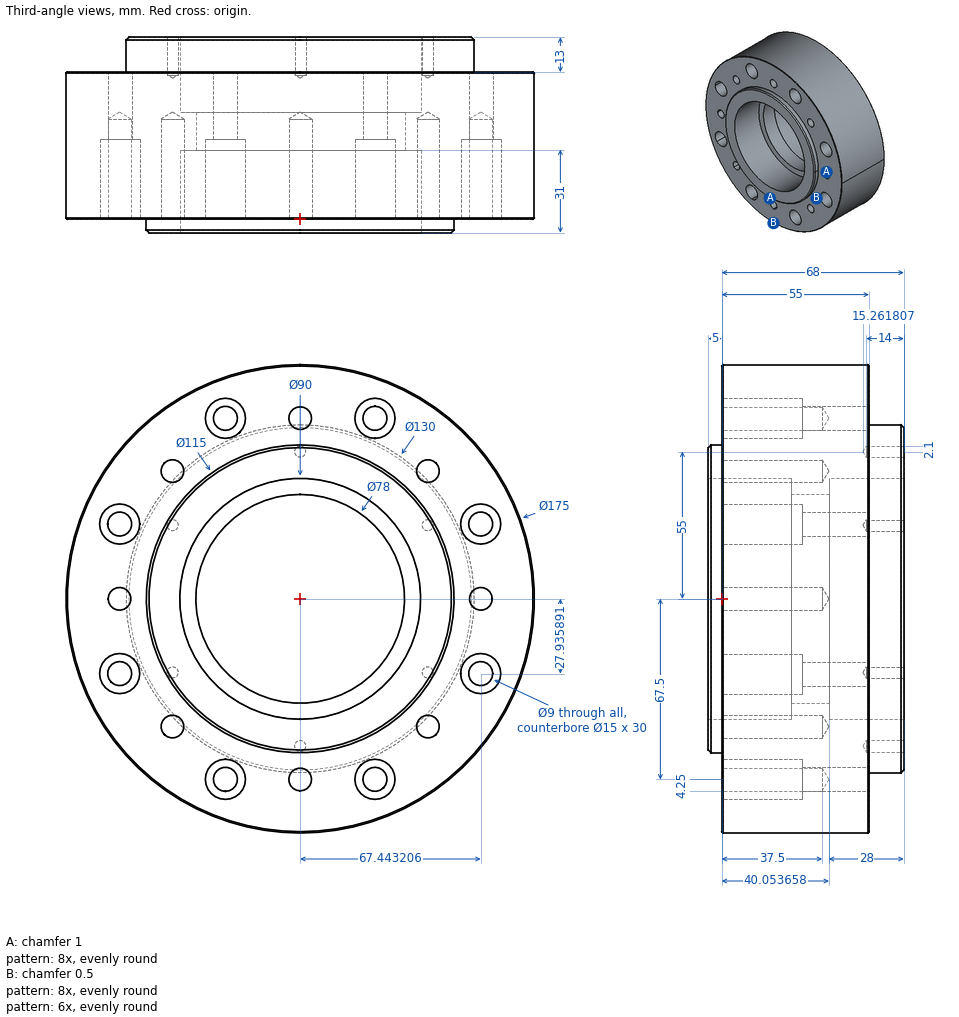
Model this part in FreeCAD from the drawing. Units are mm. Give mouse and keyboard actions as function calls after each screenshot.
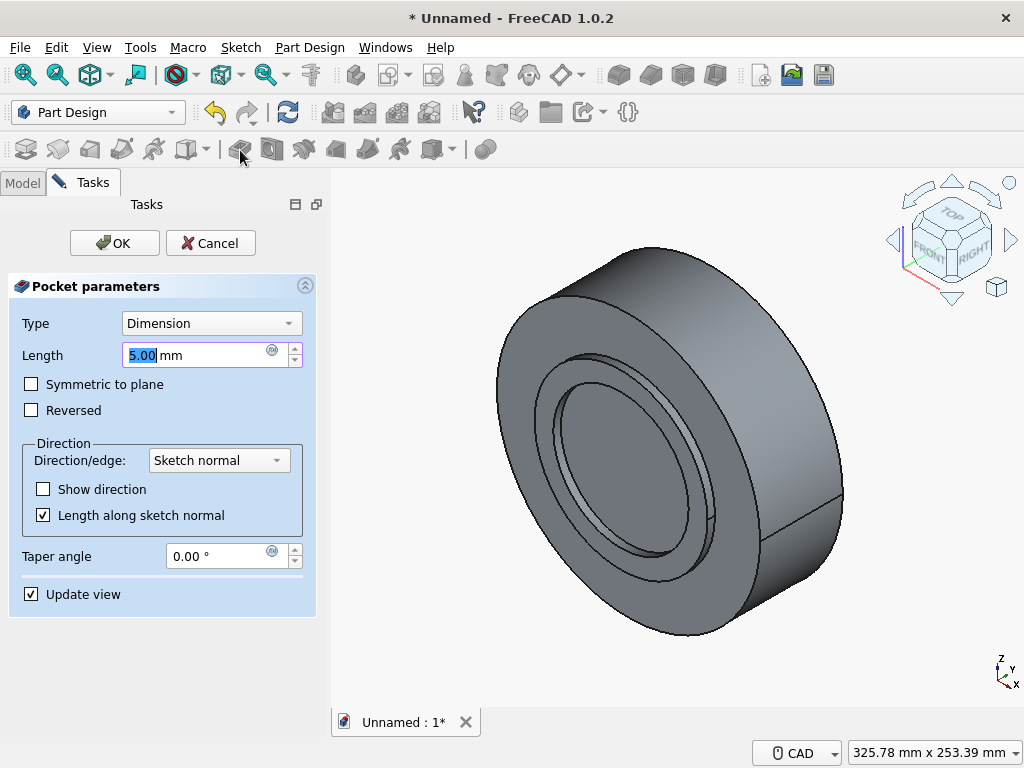
text(31)
key(Tab)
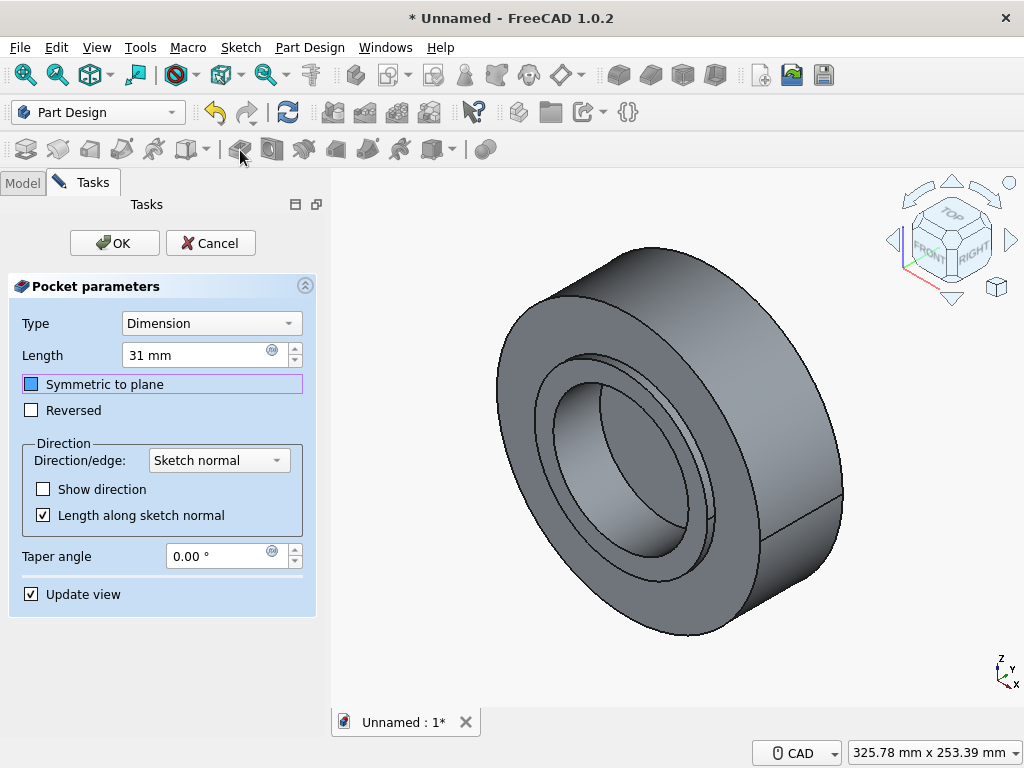
click(115, 243)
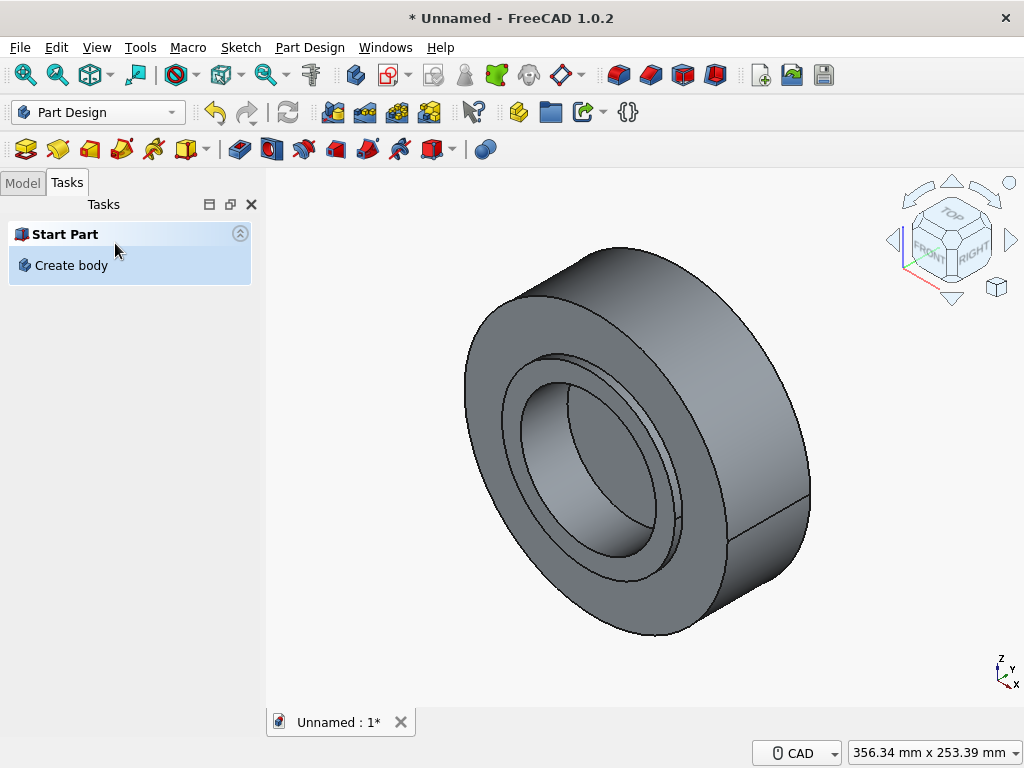
click(23, 182)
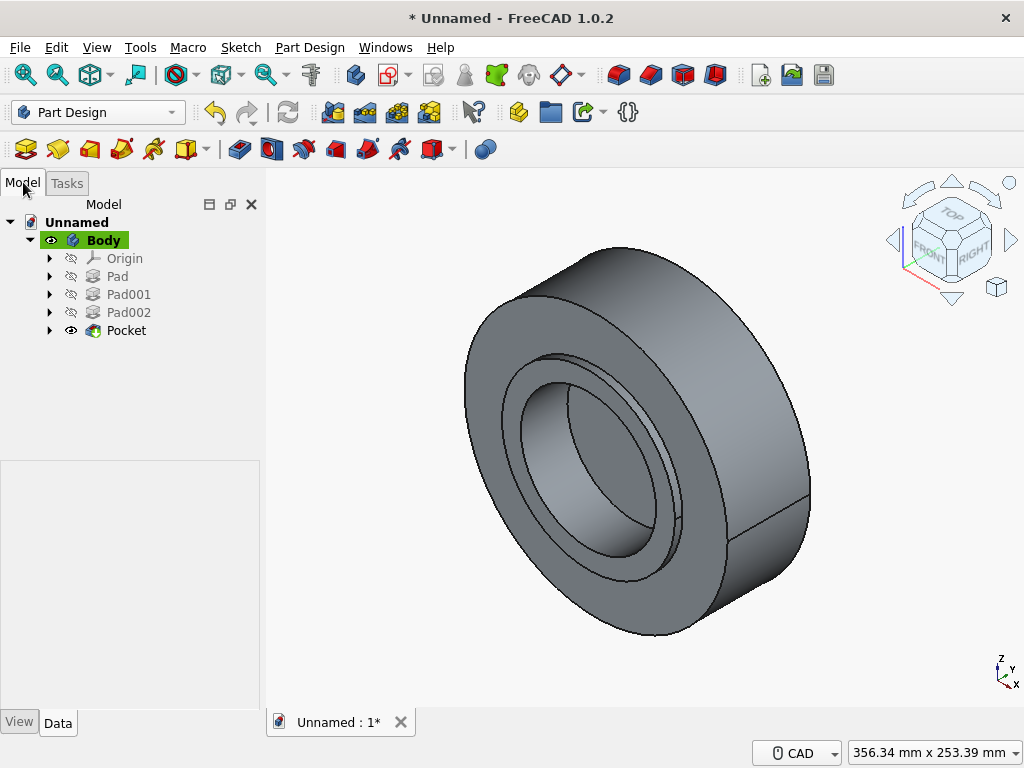
click(50, 258)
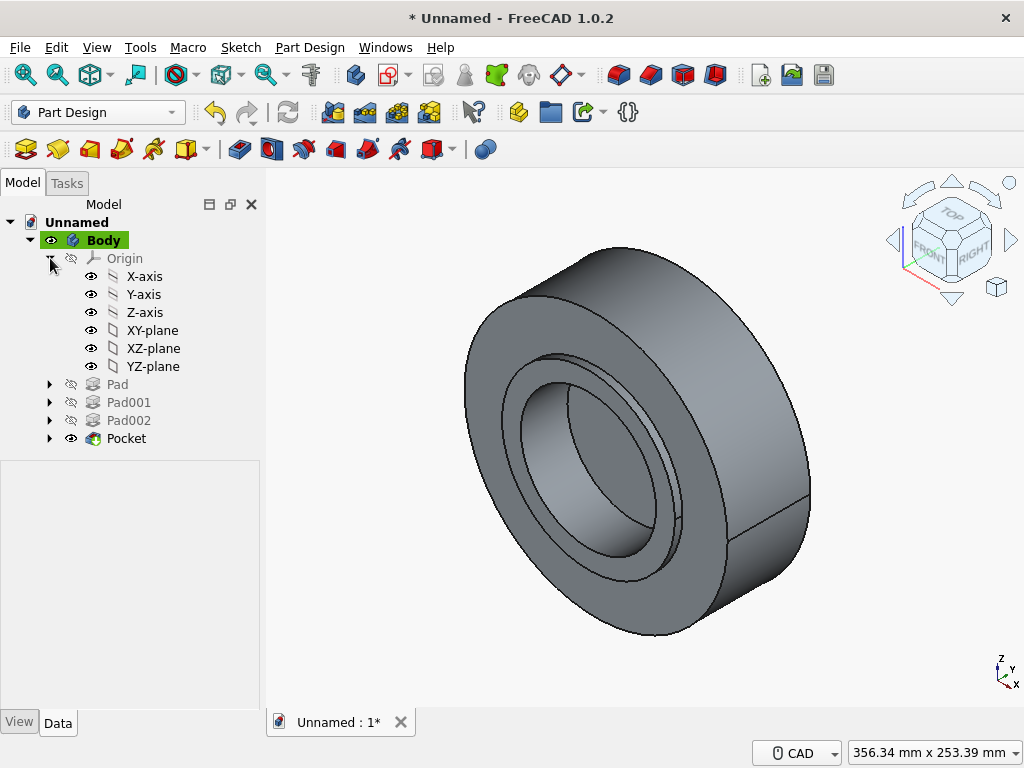
click(136, 348)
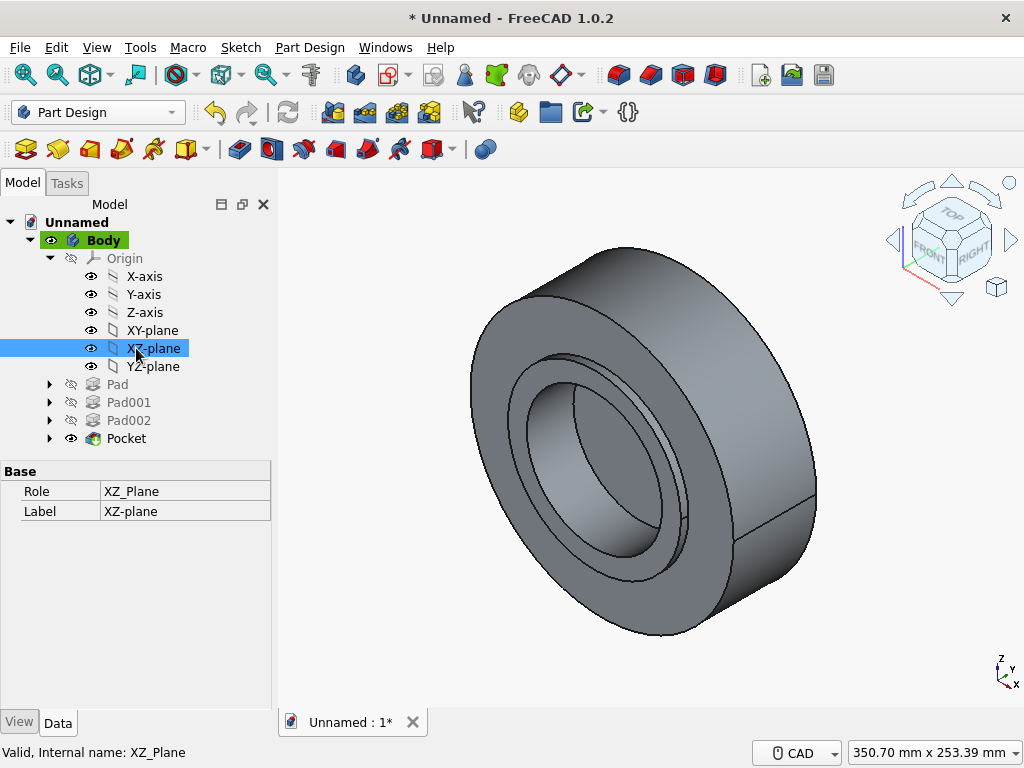
click(562, 76)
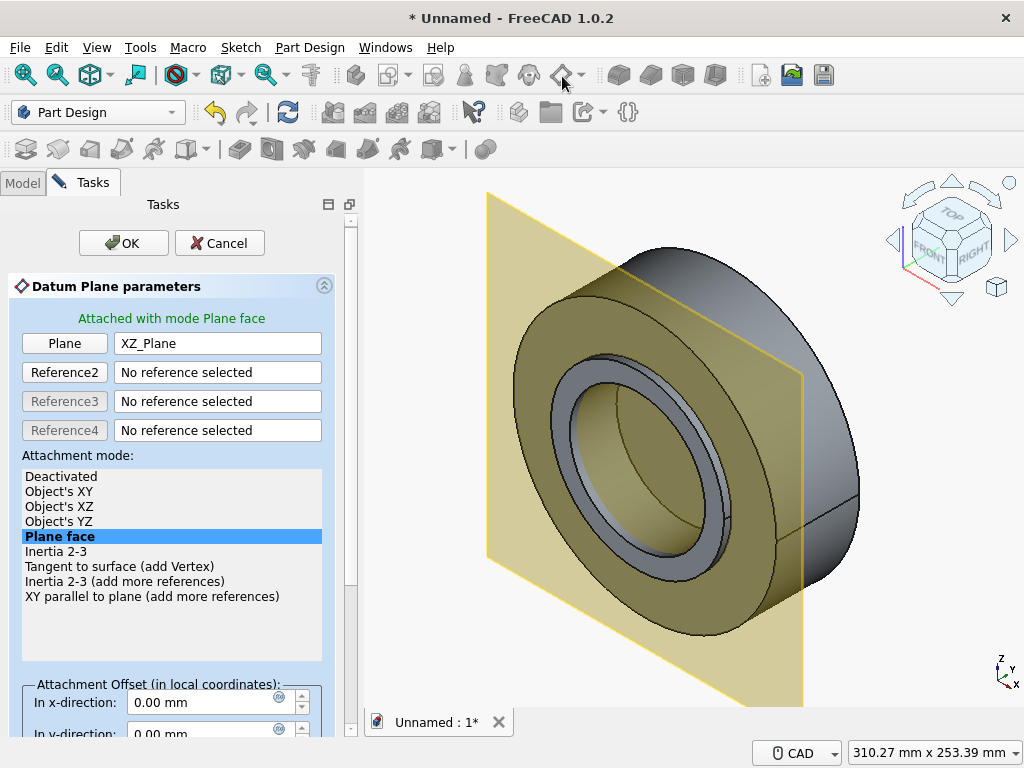
scroll(351, 475, down, 2)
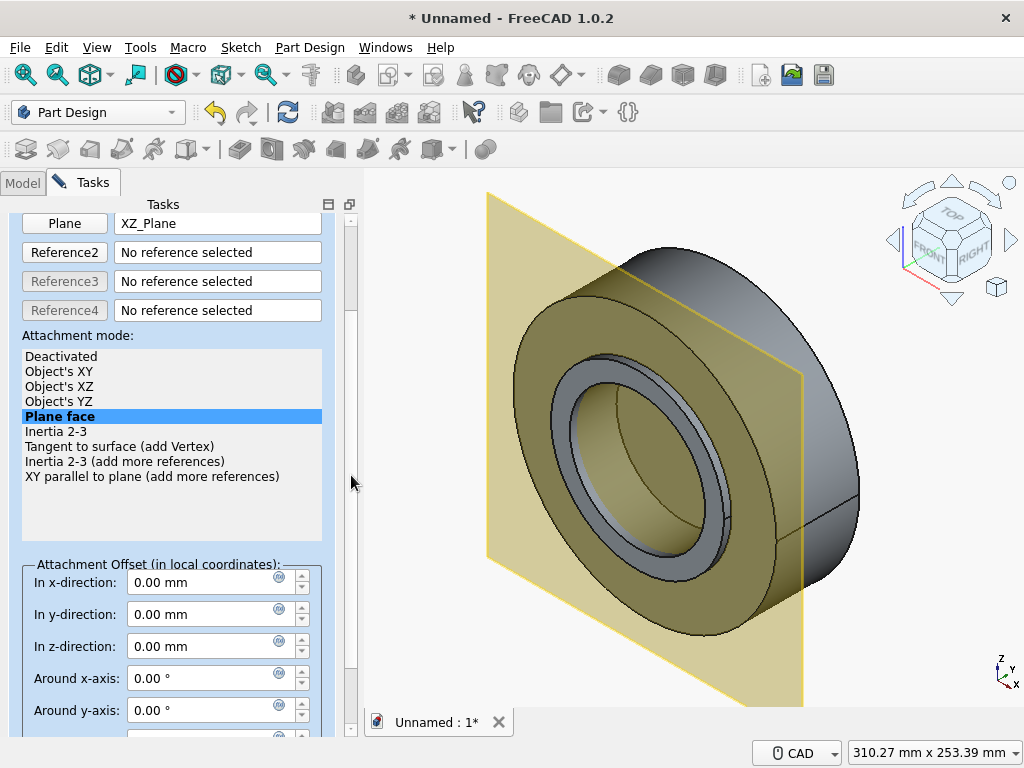
triple_click(210, 646)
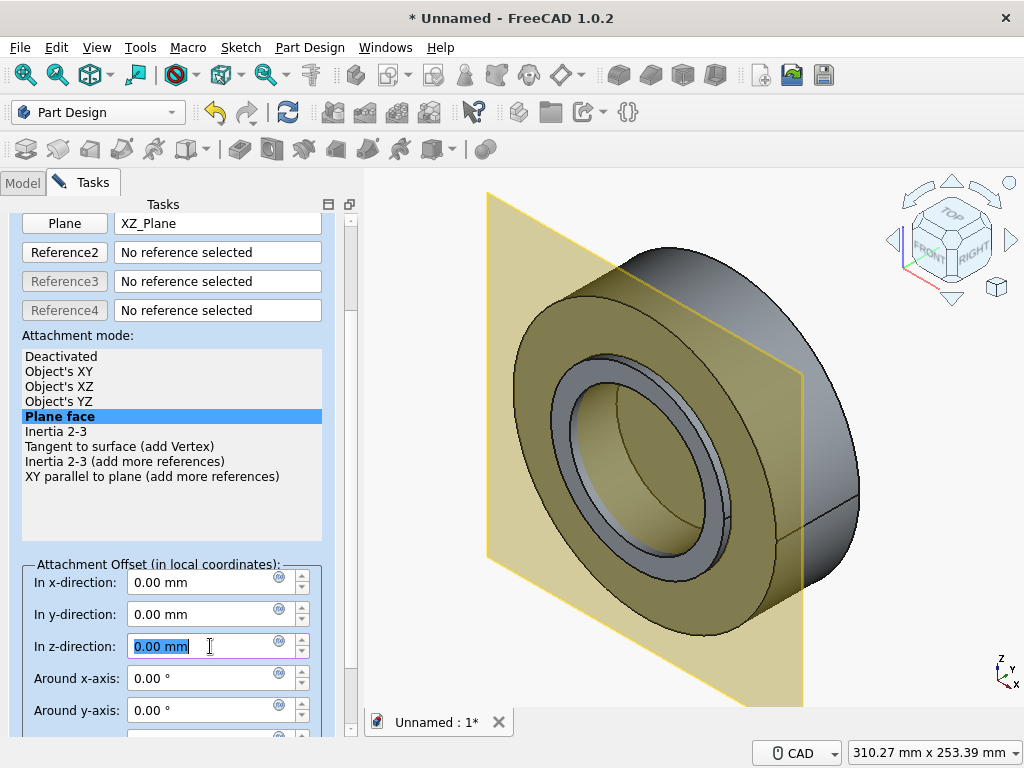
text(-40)
key(Tab)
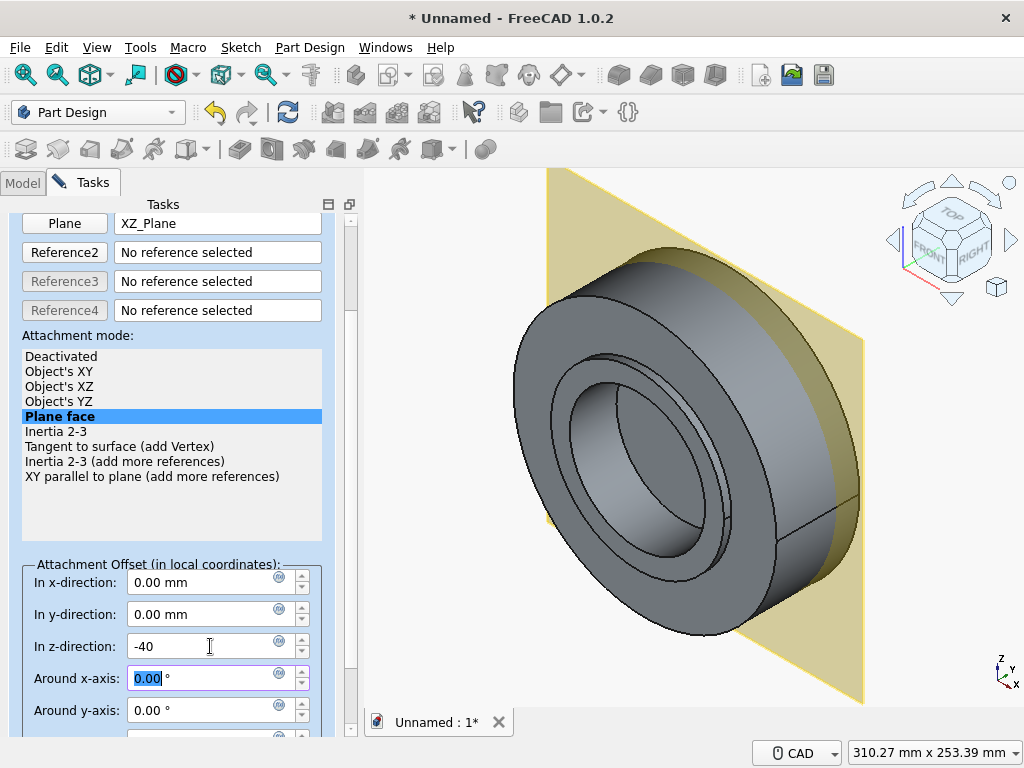
scroll(351, 475, up, 3)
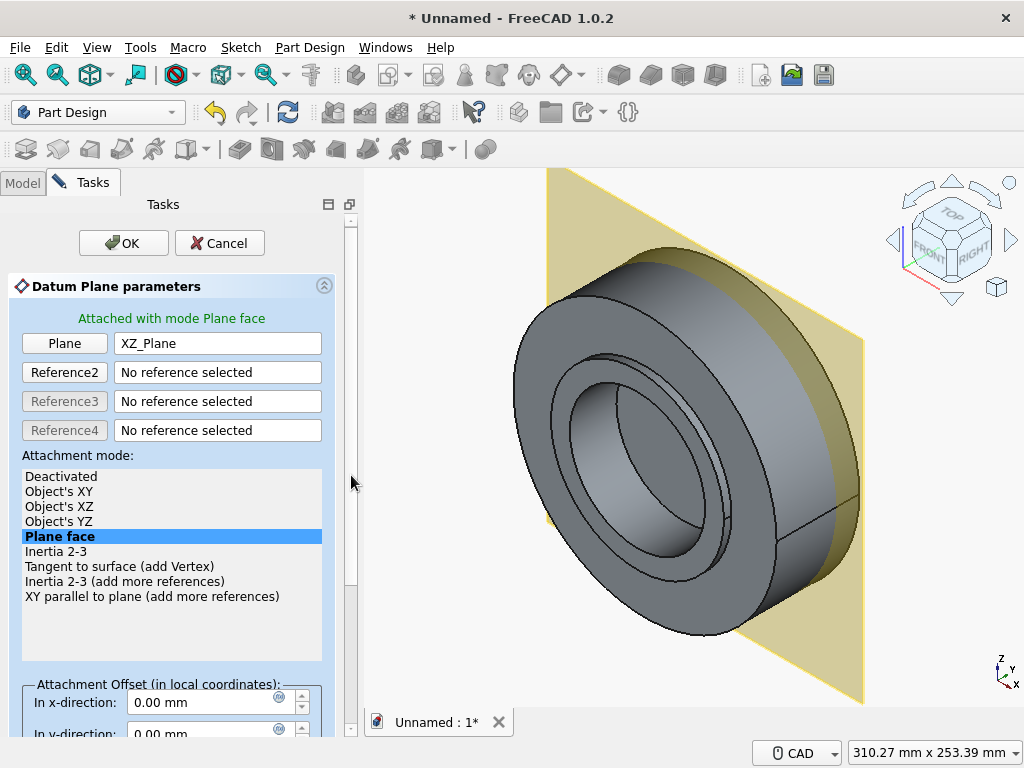
click(124, 243)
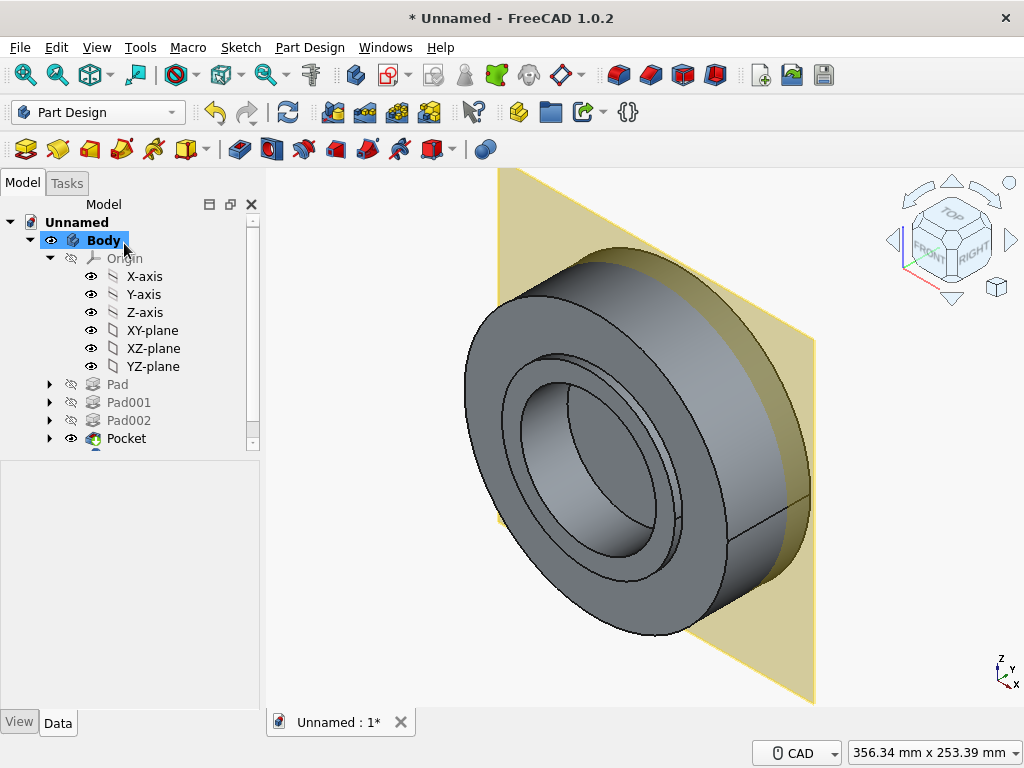
scroll(100, 326, down, 3)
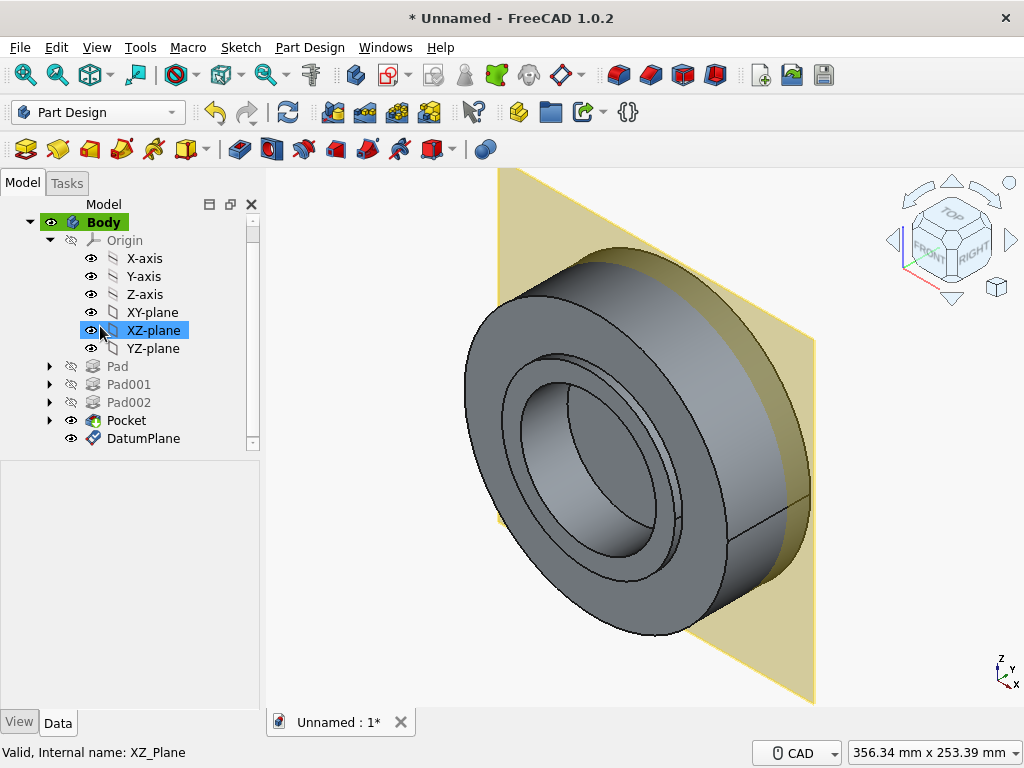
click(116, 438)